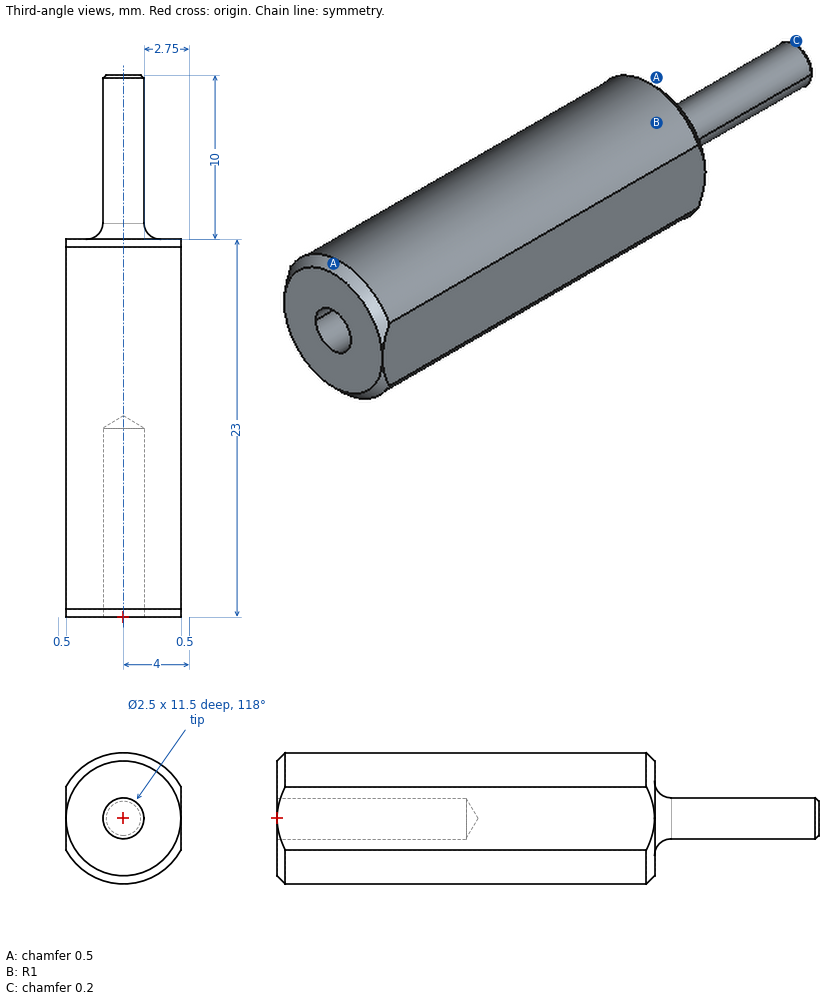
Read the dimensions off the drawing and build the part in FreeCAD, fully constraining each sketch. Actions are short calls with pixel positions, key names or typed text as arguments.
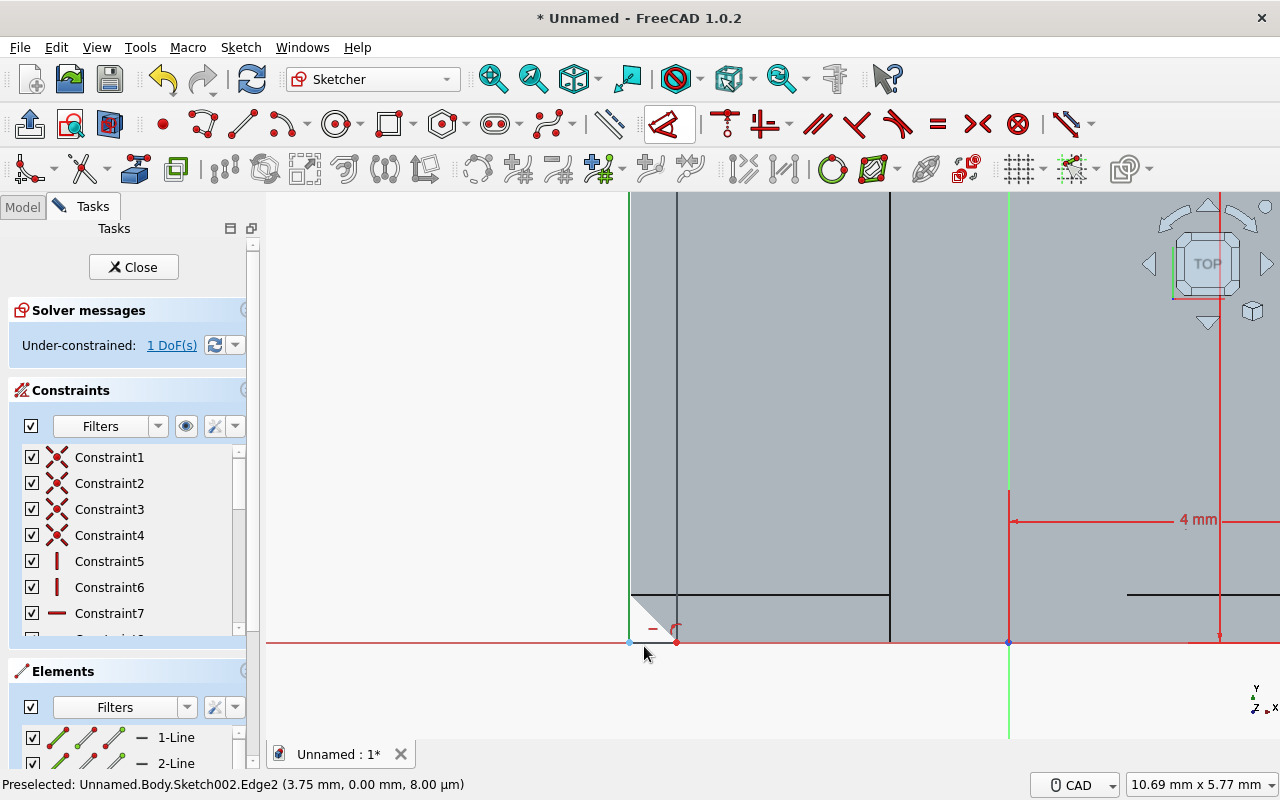
click(644, 643)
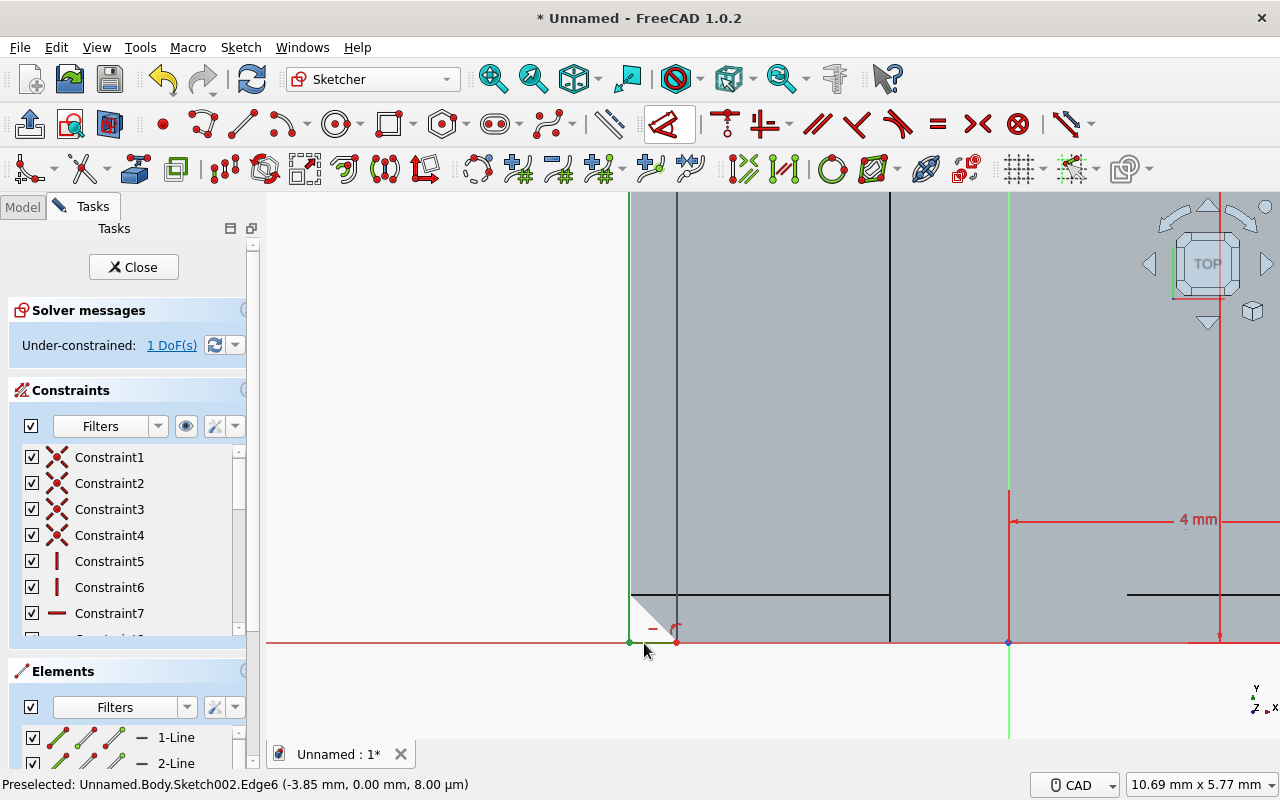
key(l)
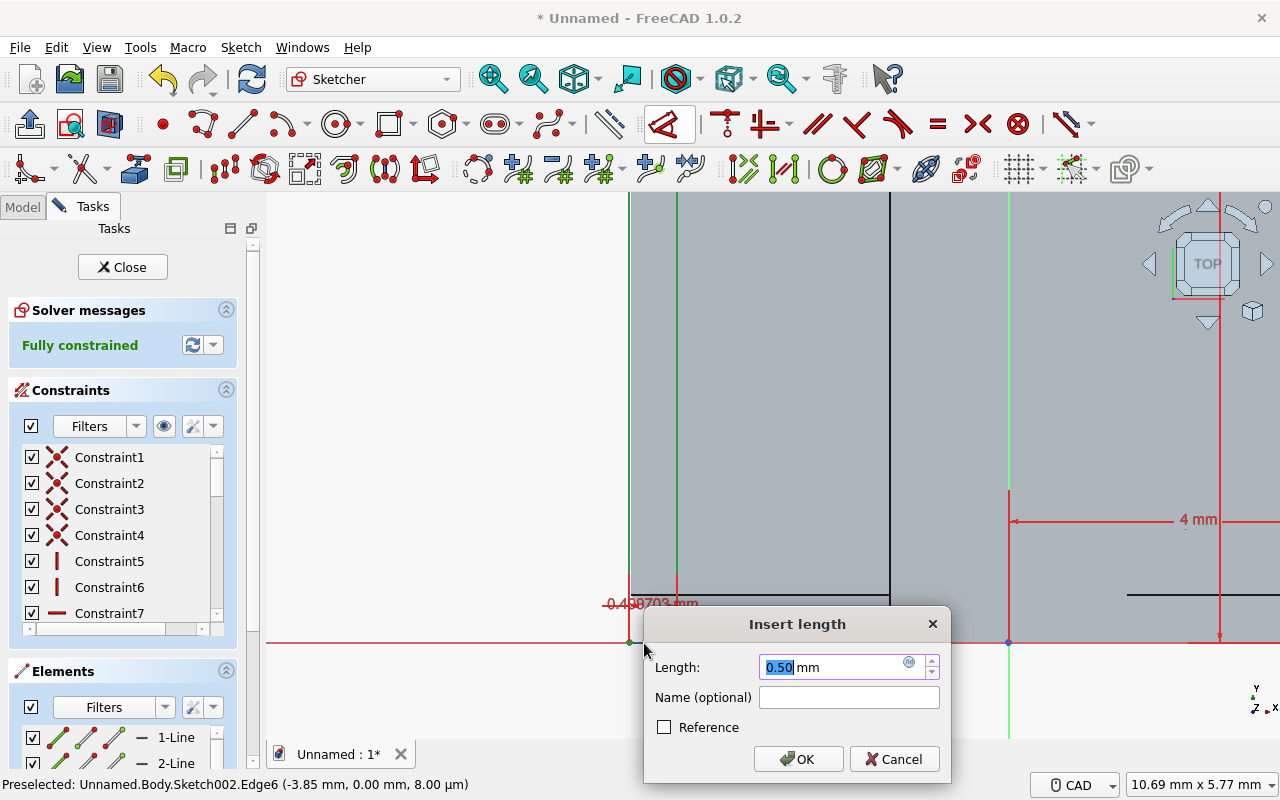
text(0.5)
key(Return)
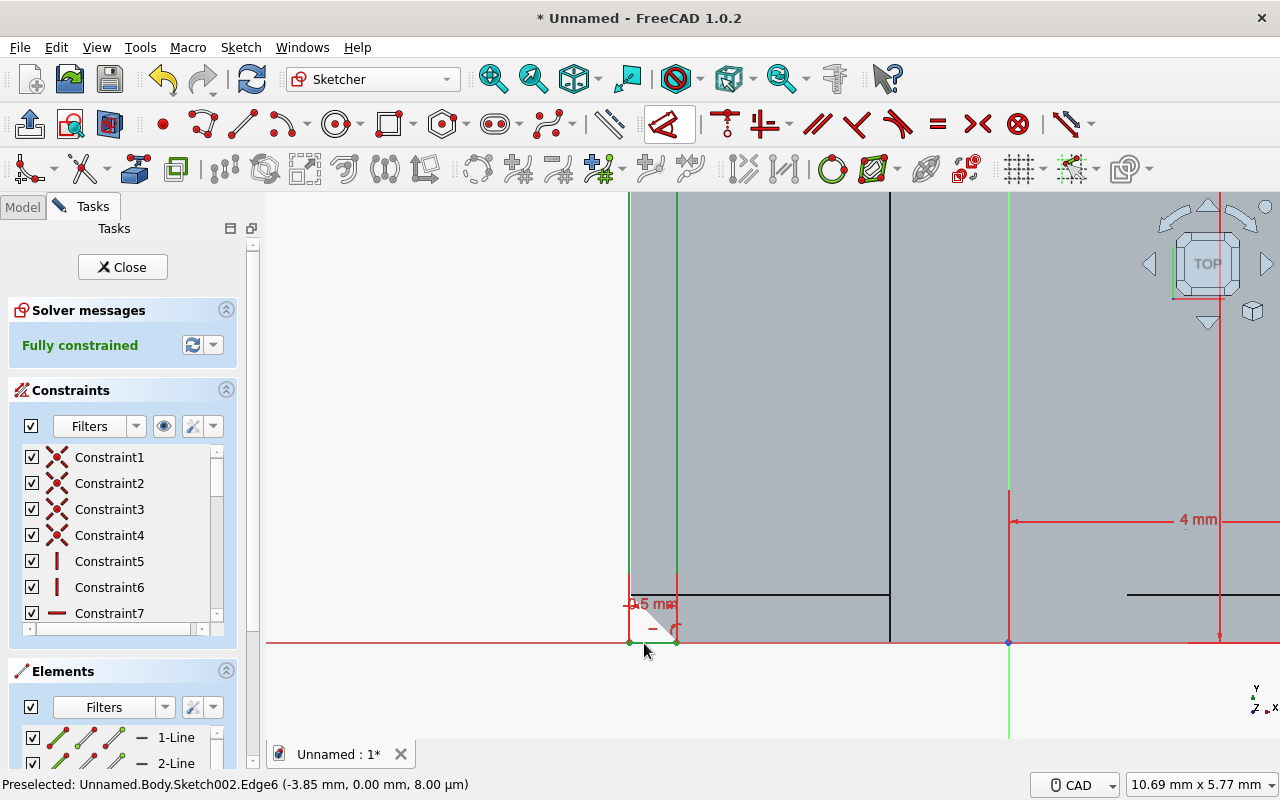
click(123, 267)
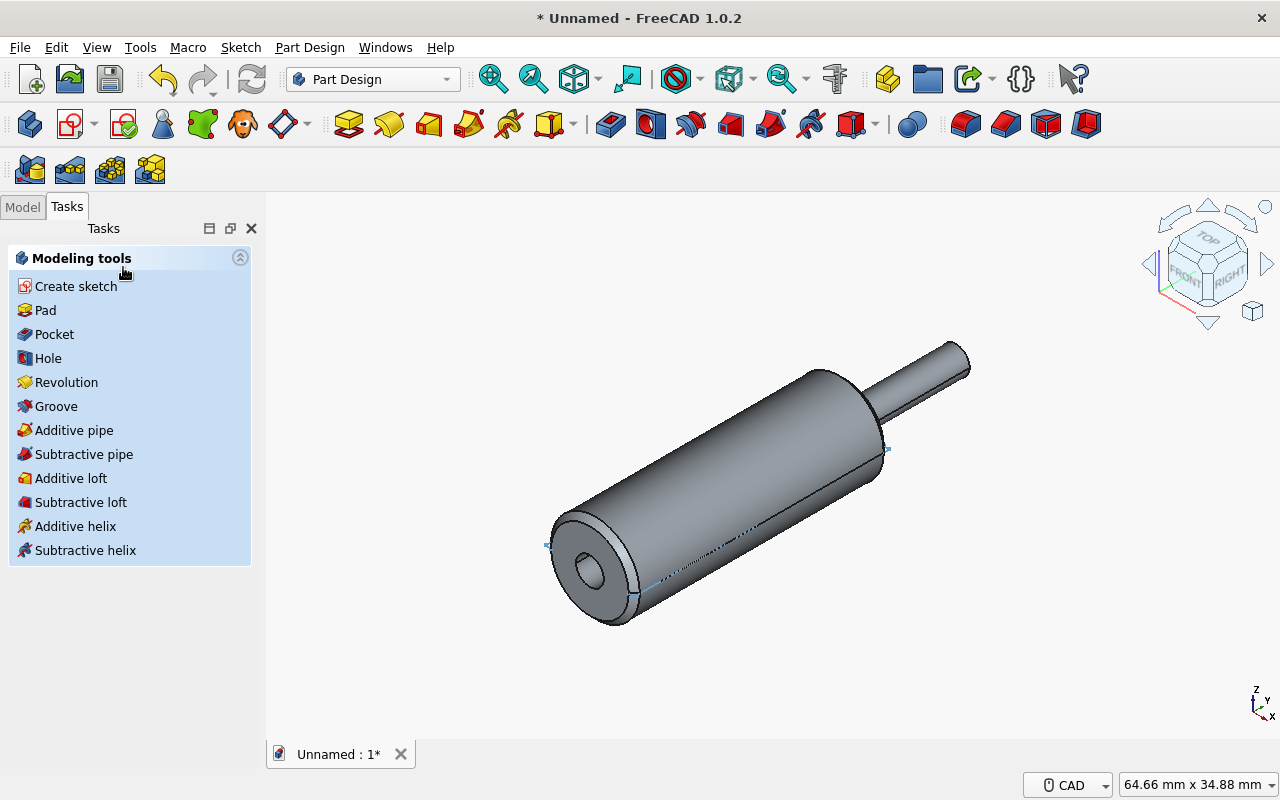
click(612, 124)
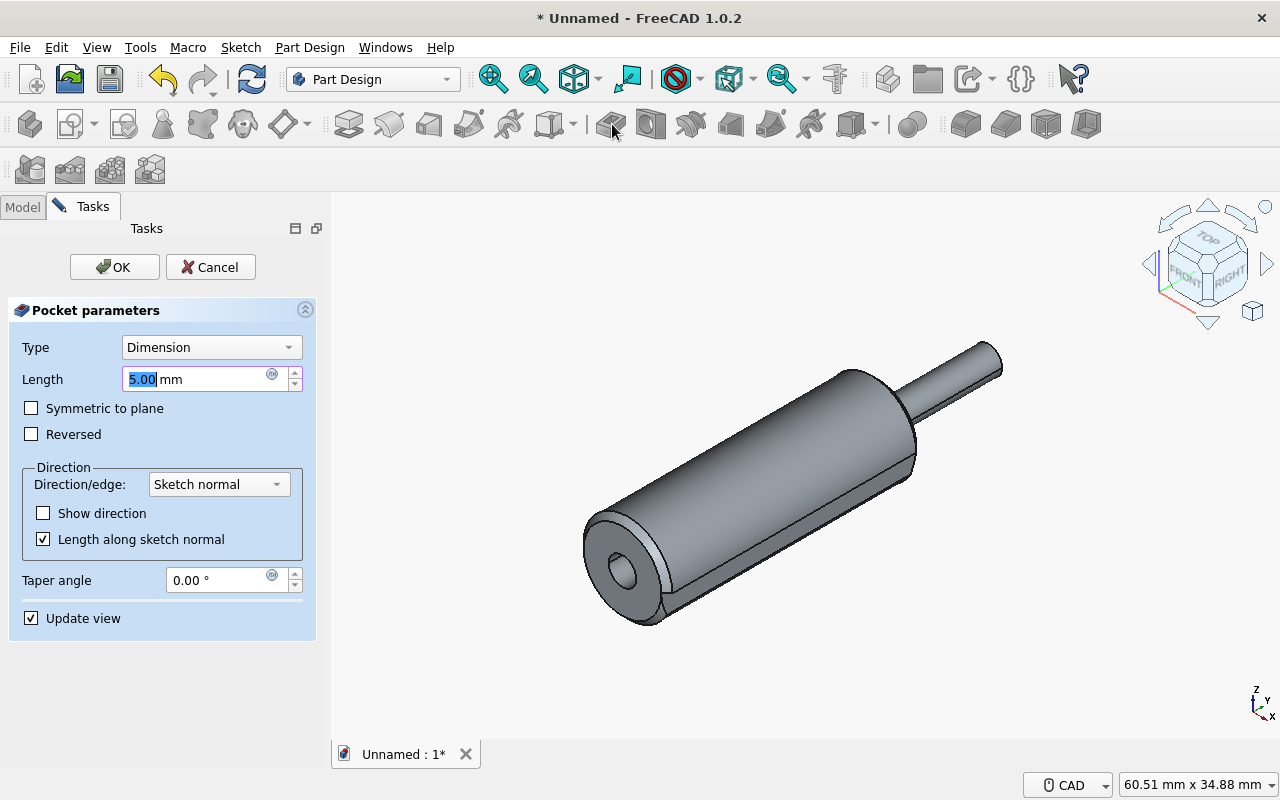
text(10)
key(Tab)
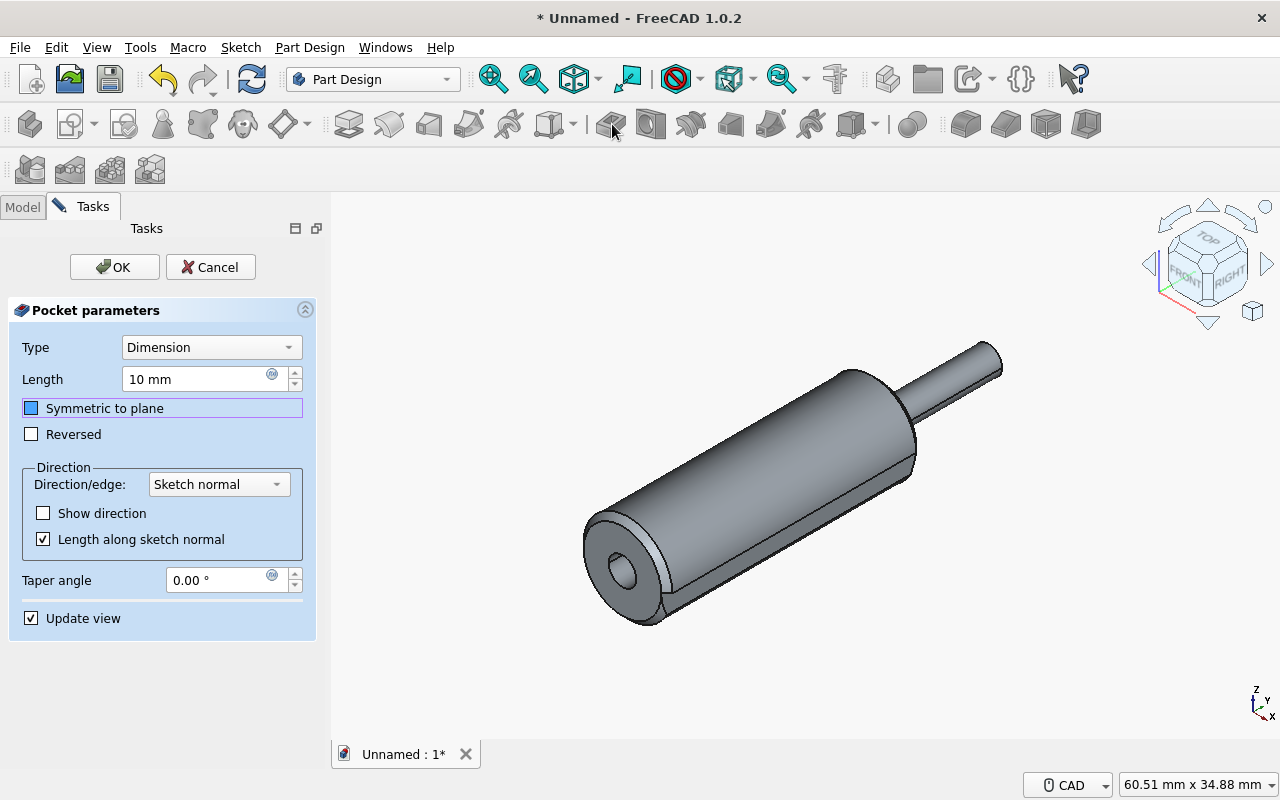
click(30, 408)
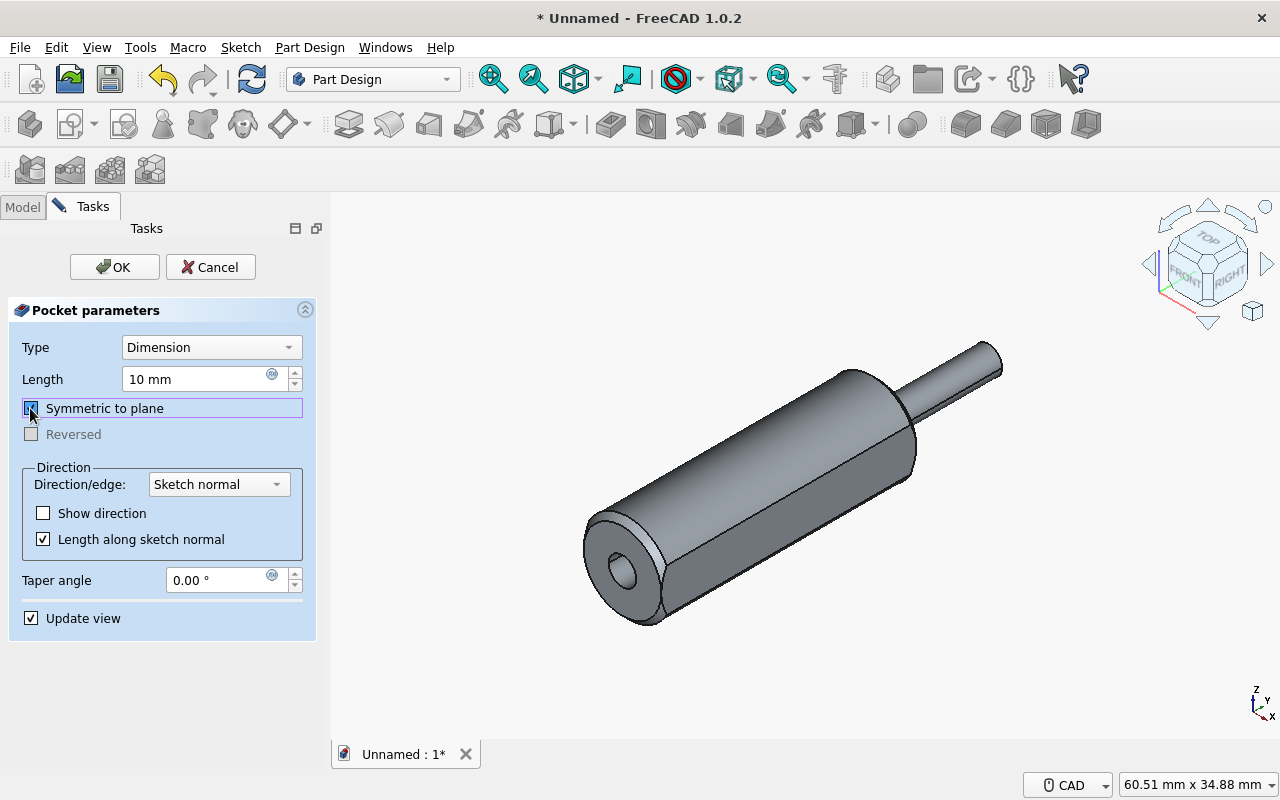
click(115, 267)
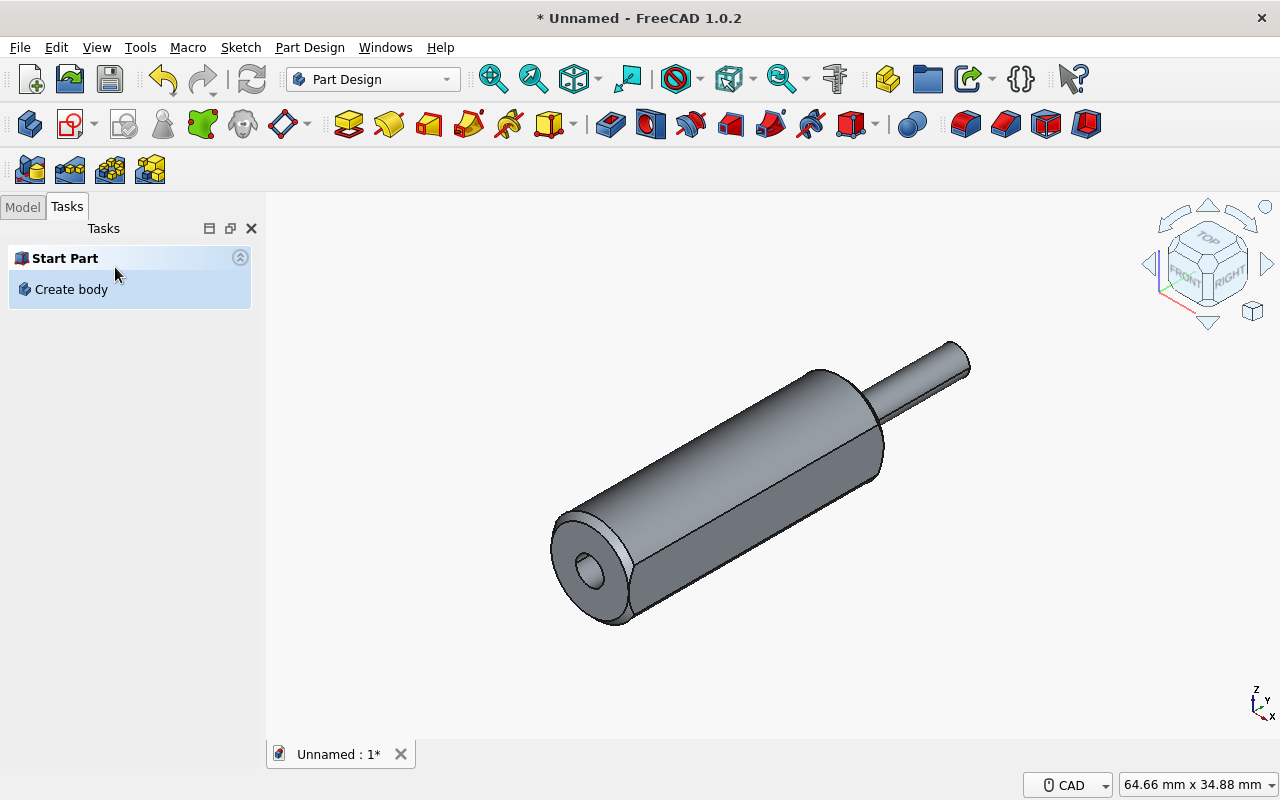
click(952, 341)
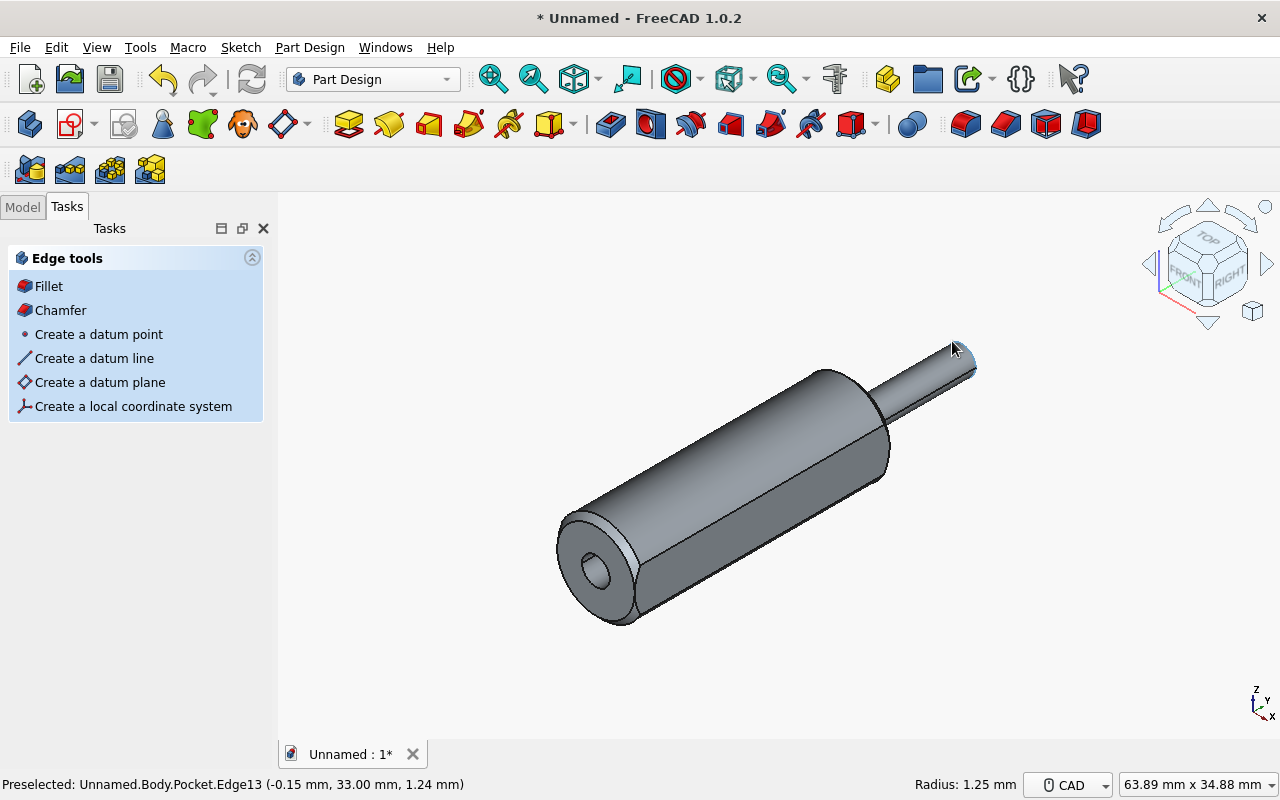
click(1006, 124)